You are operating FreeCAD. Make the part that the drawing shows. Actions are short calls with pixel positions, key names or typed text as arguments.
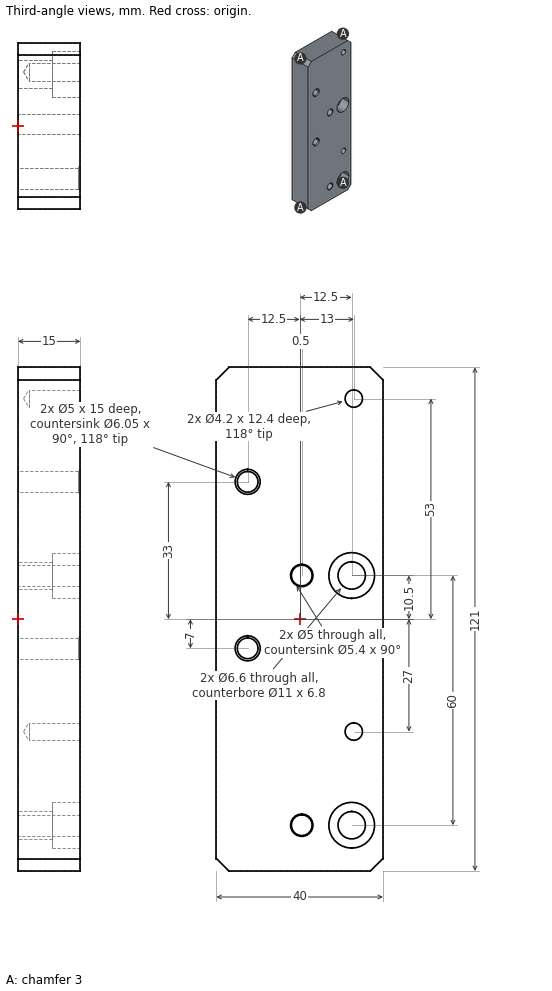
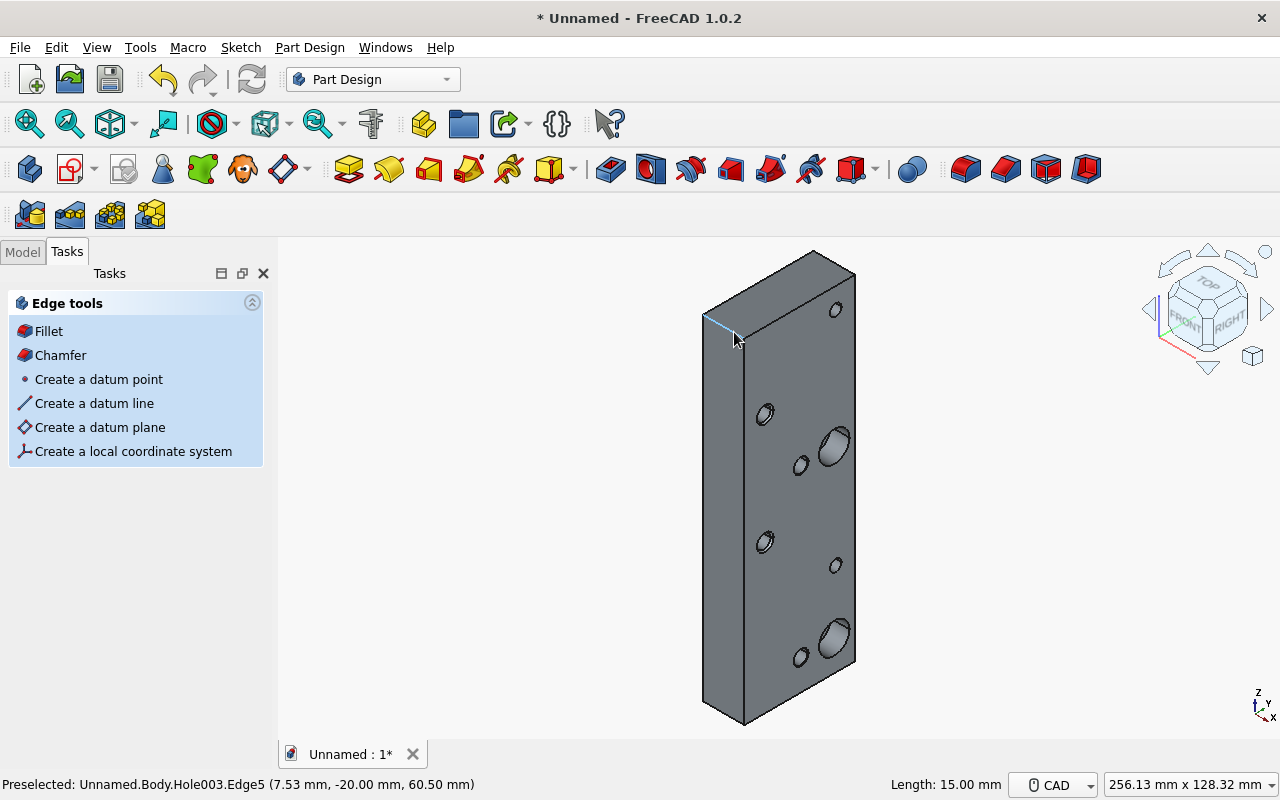
key(2)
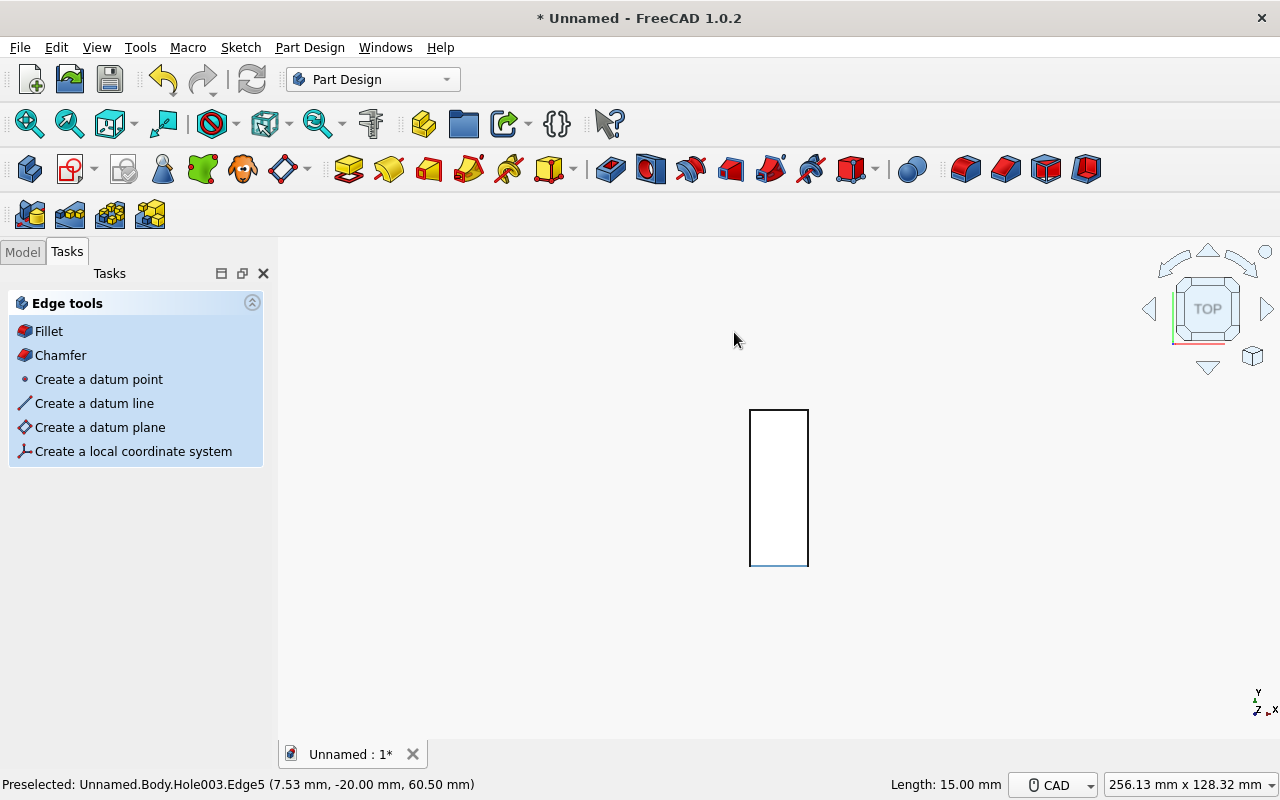
click(30, 124)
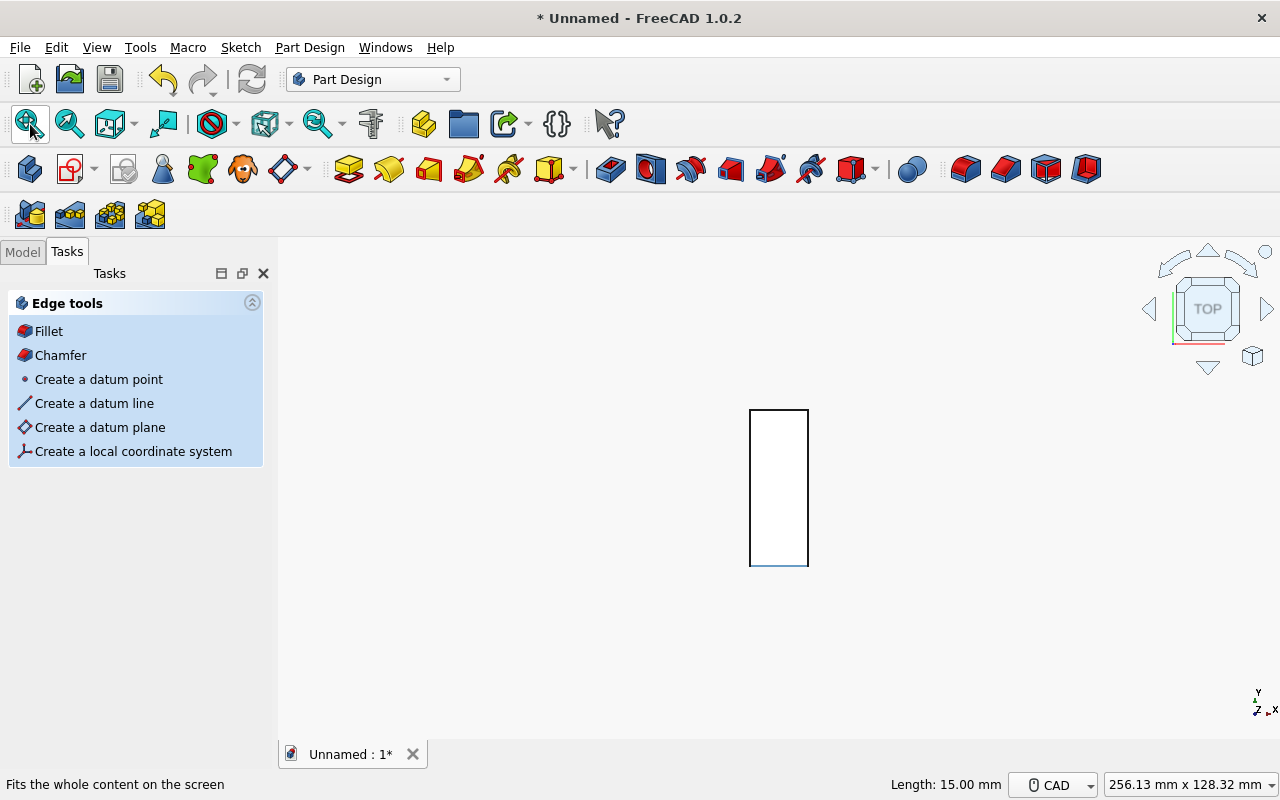
click(779, 409, ctrl)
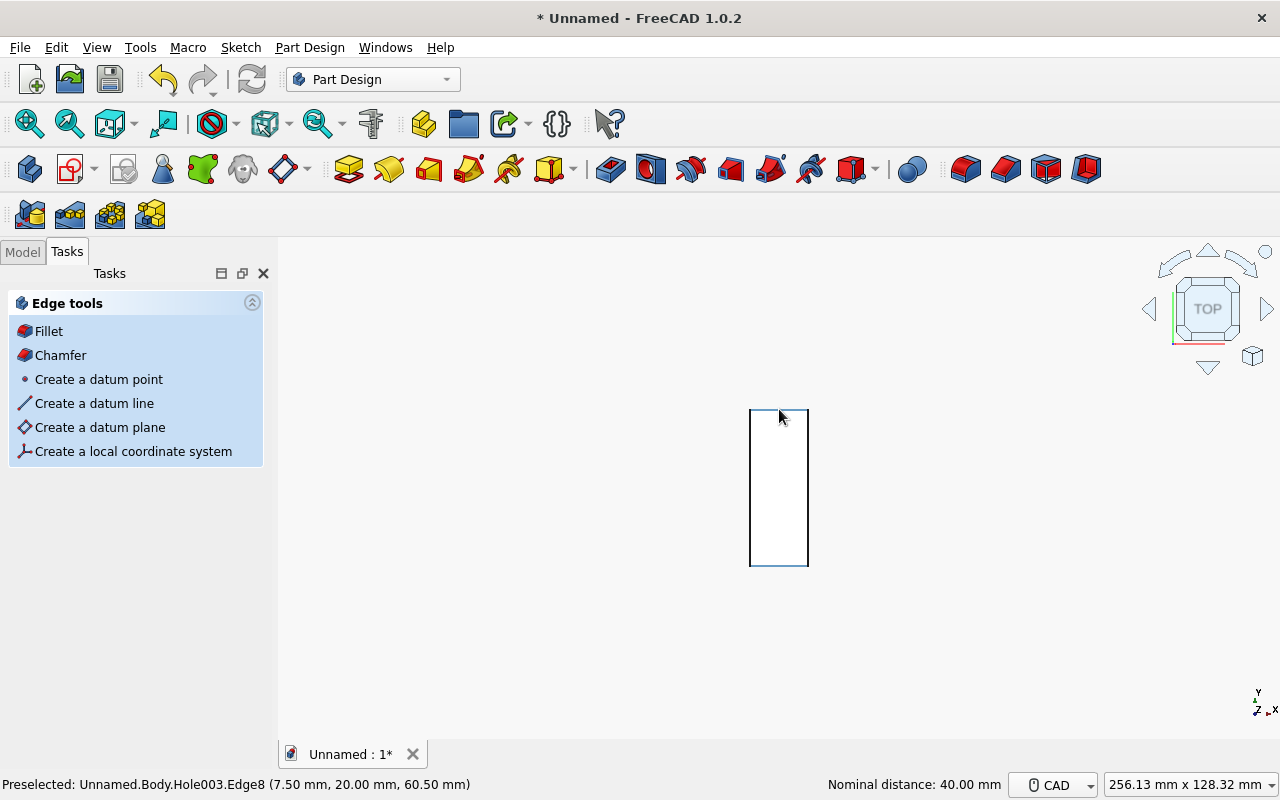
key(1)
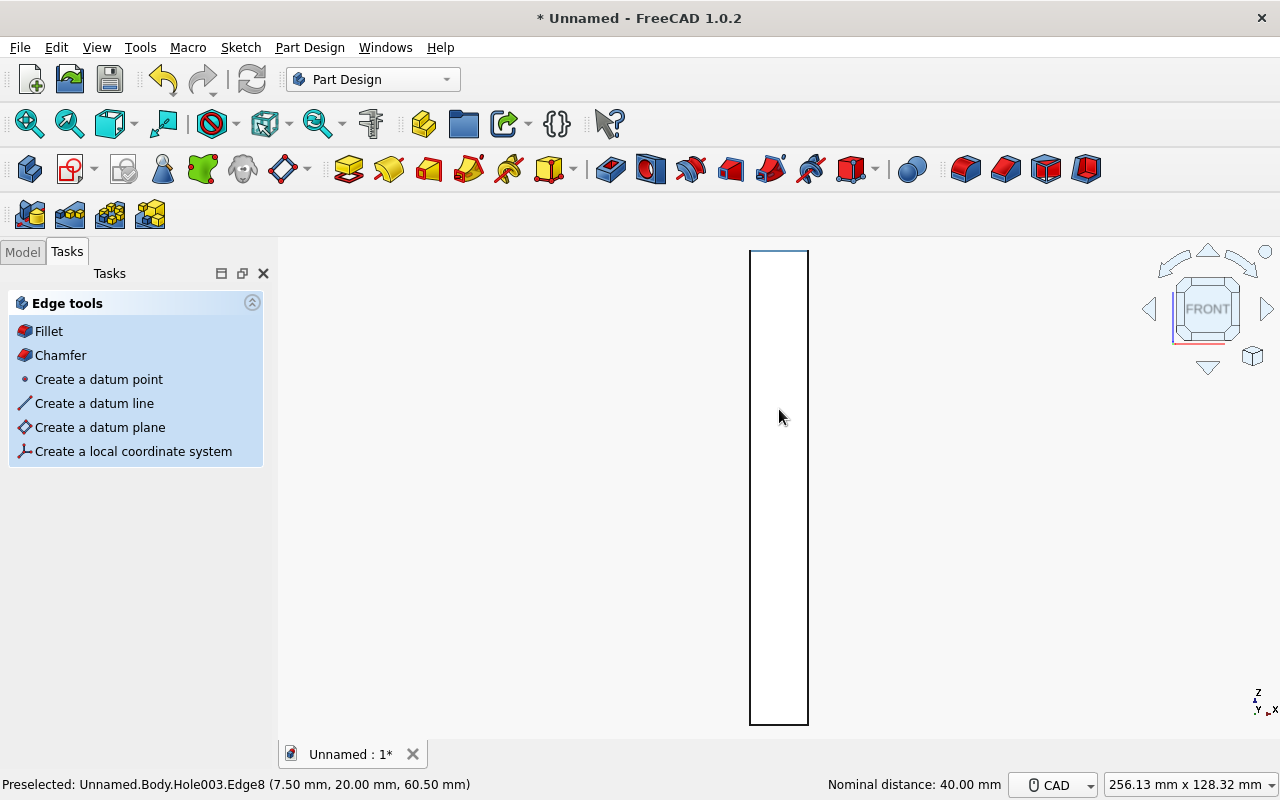
key(3)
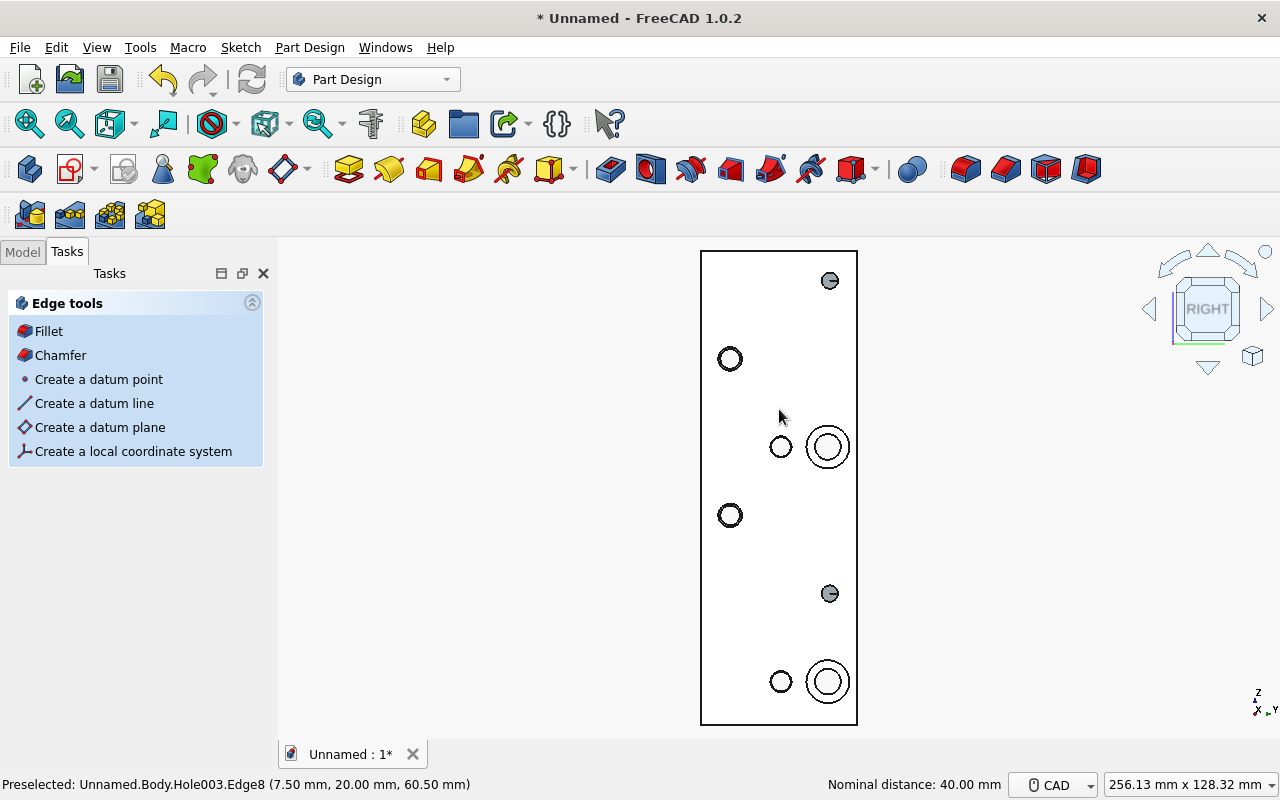
key(5)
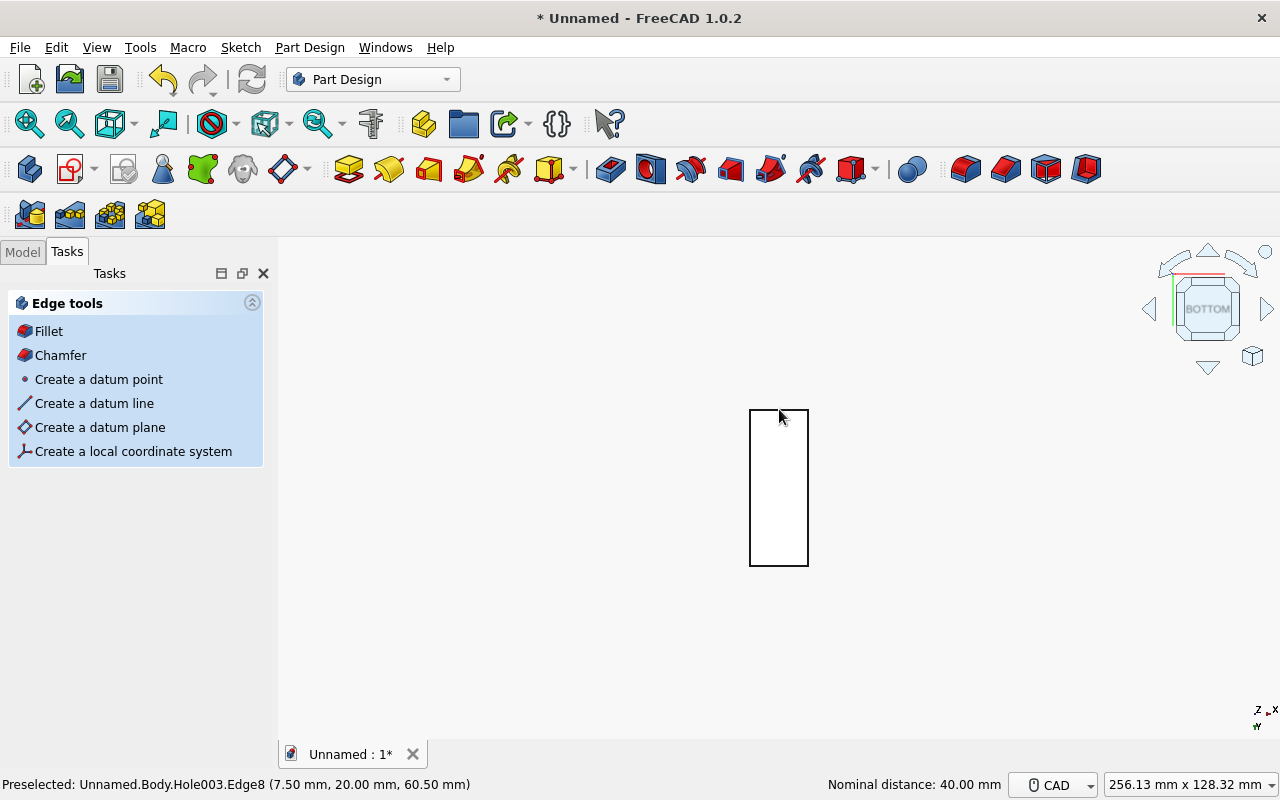
click(30, 124)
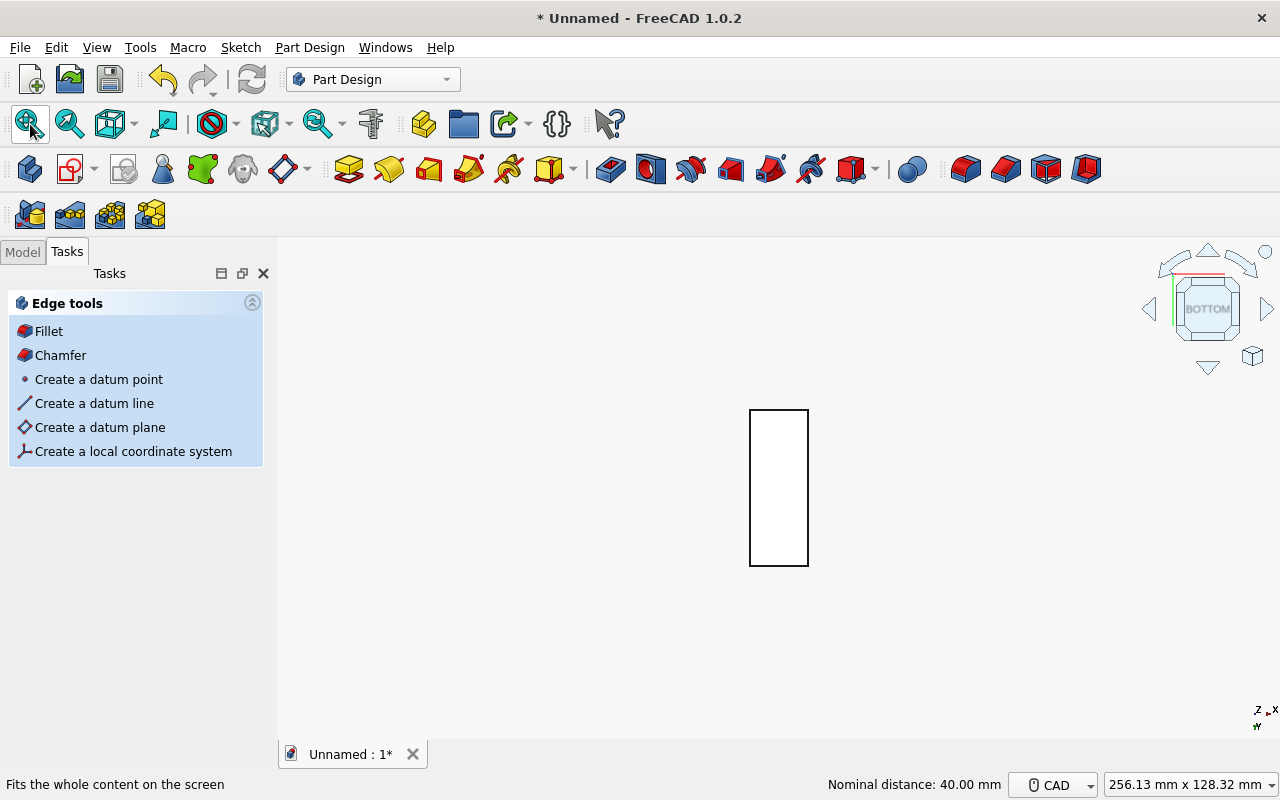
click(779, 409, ctrl)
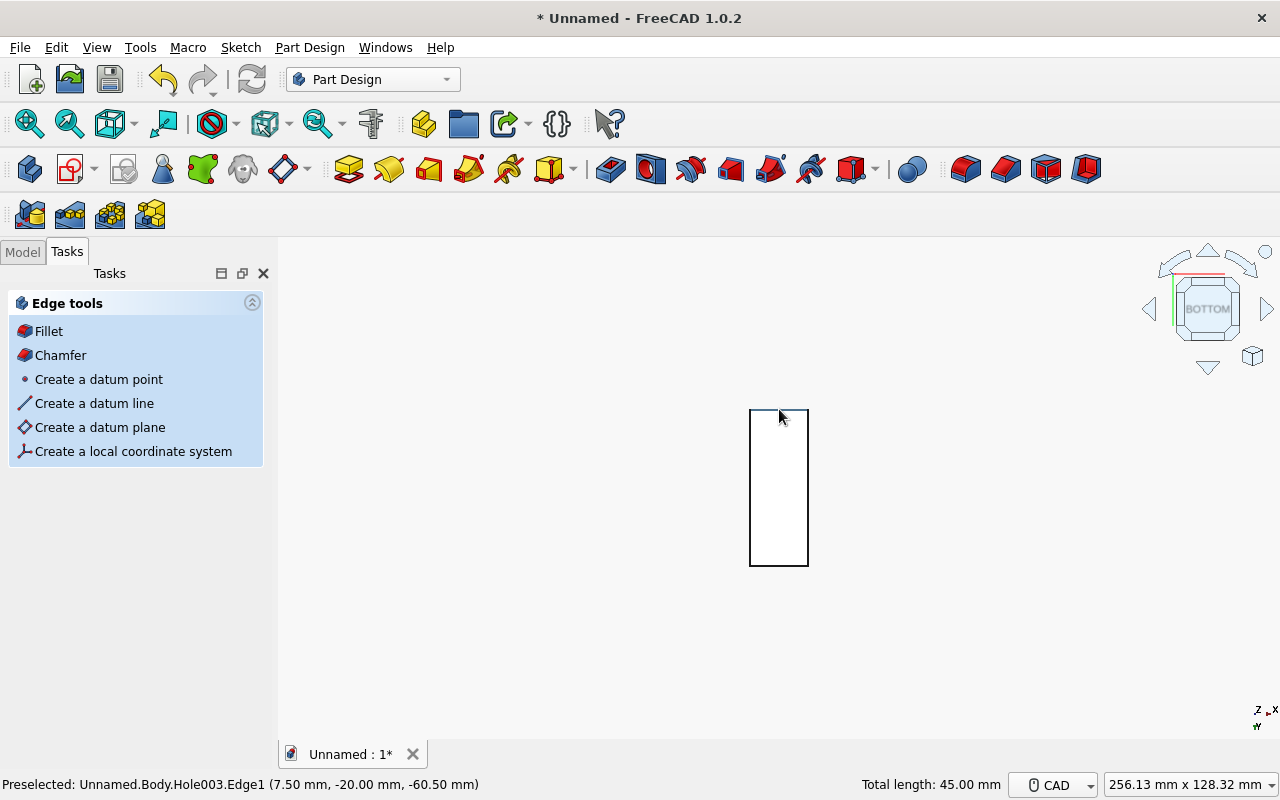
click(779, 565, ctrl)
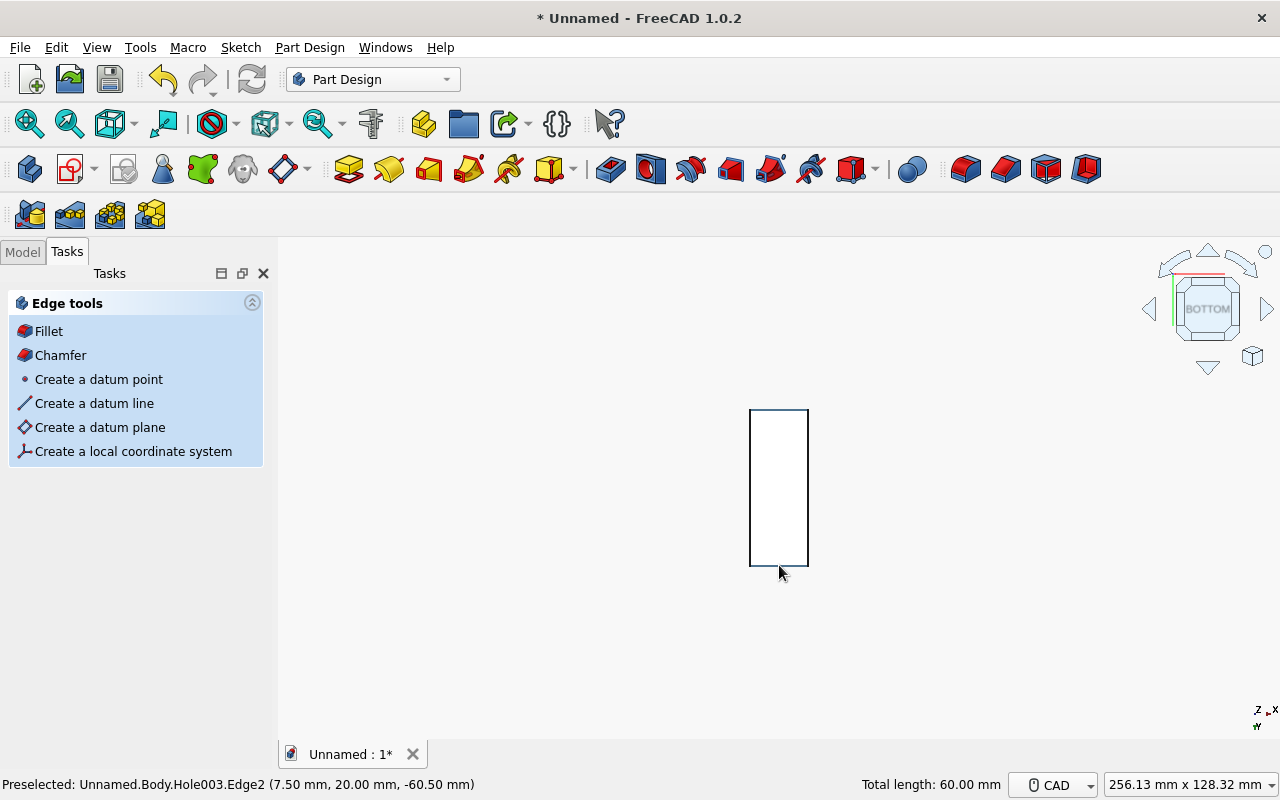
click(1006, 170)